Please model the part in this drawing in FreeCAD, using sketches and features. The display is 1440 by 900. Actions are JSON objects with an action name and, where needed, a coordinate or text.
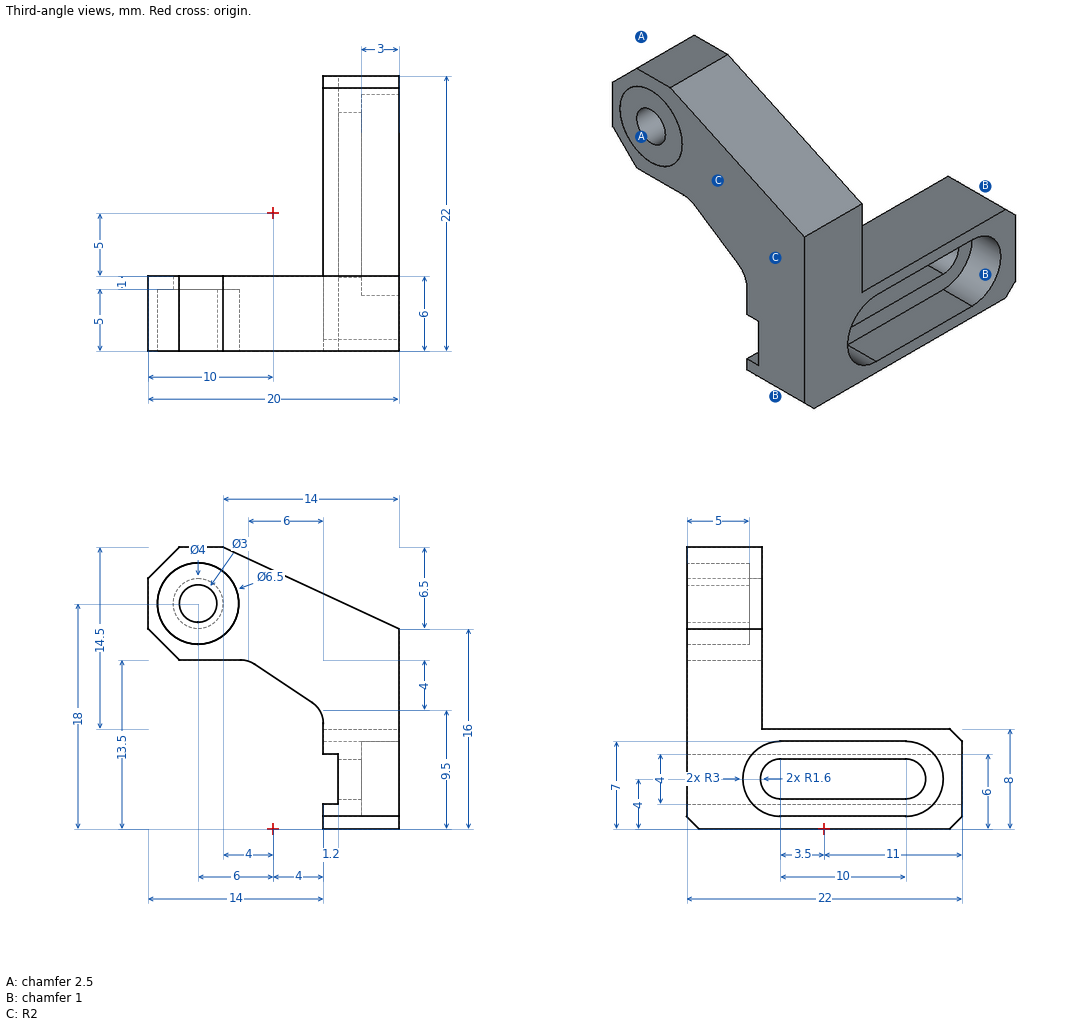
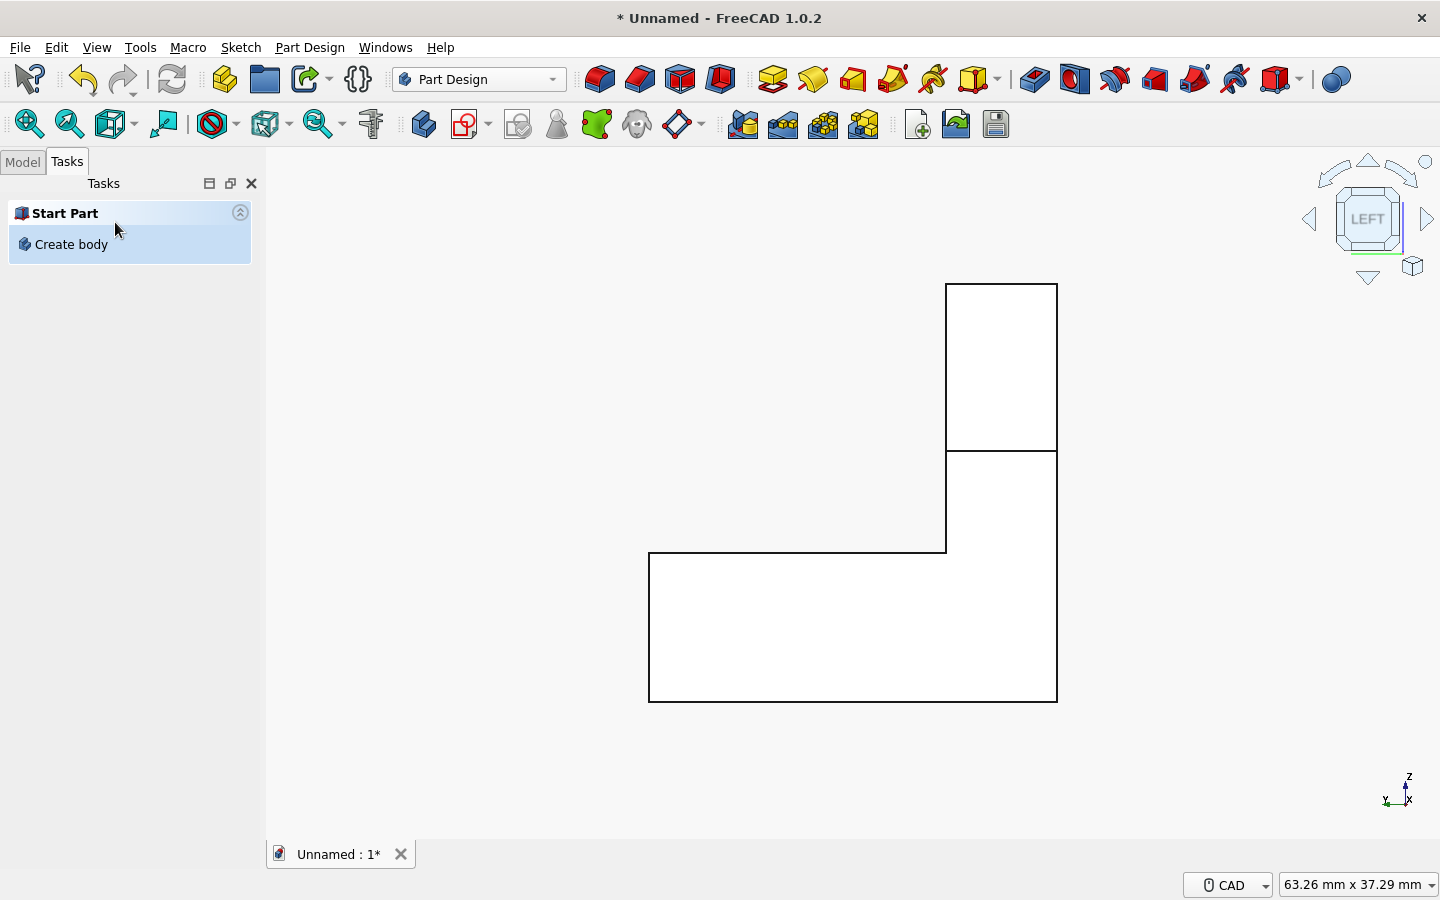
{"action": "left_click", "coordinate": [970, 611]}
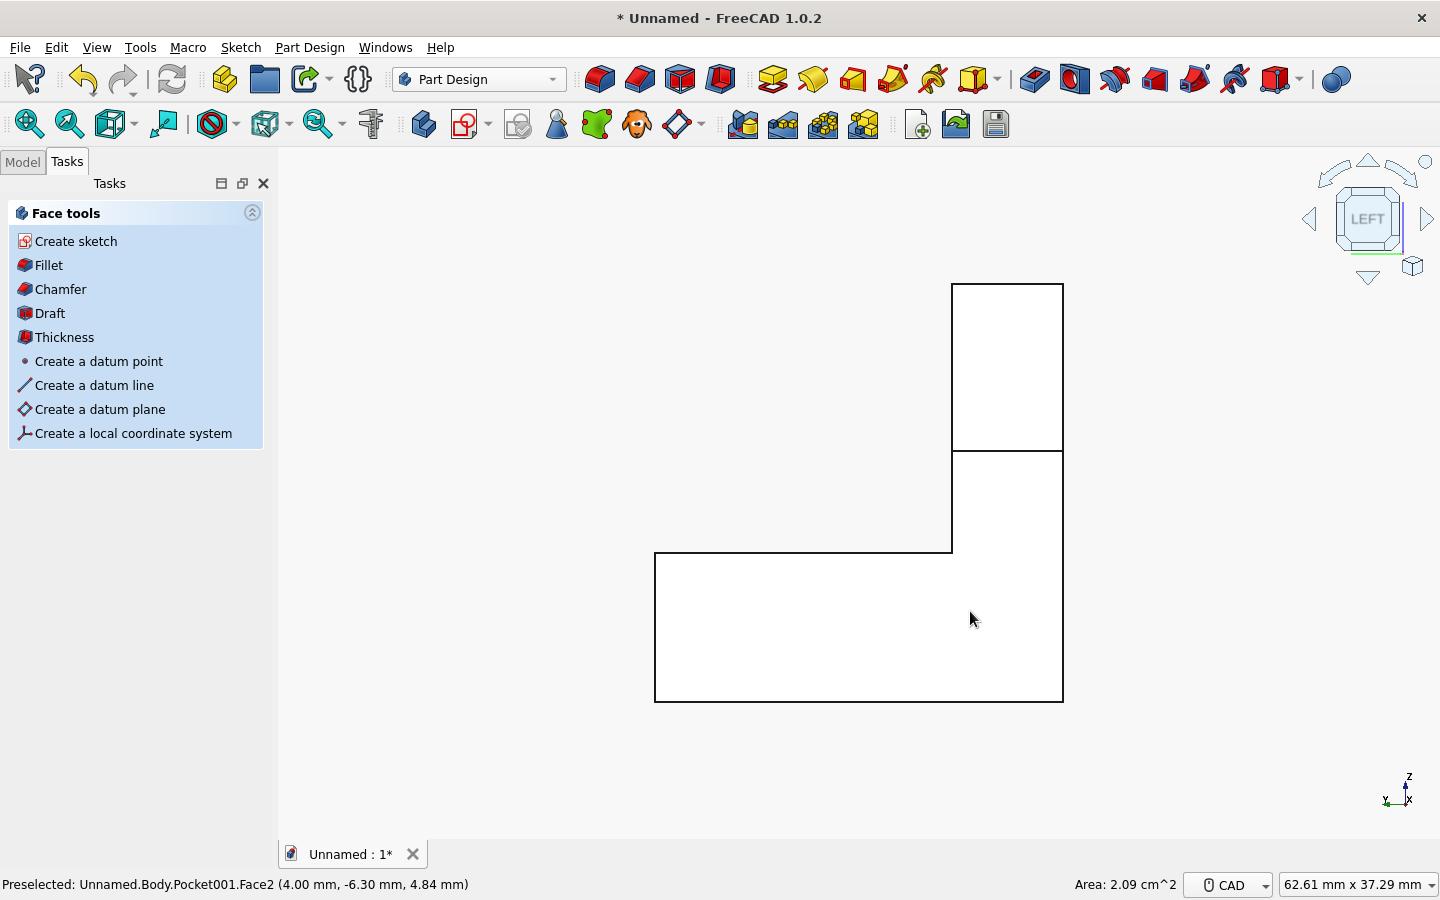
{"action": "left_click", "coordinate": [464, 124]}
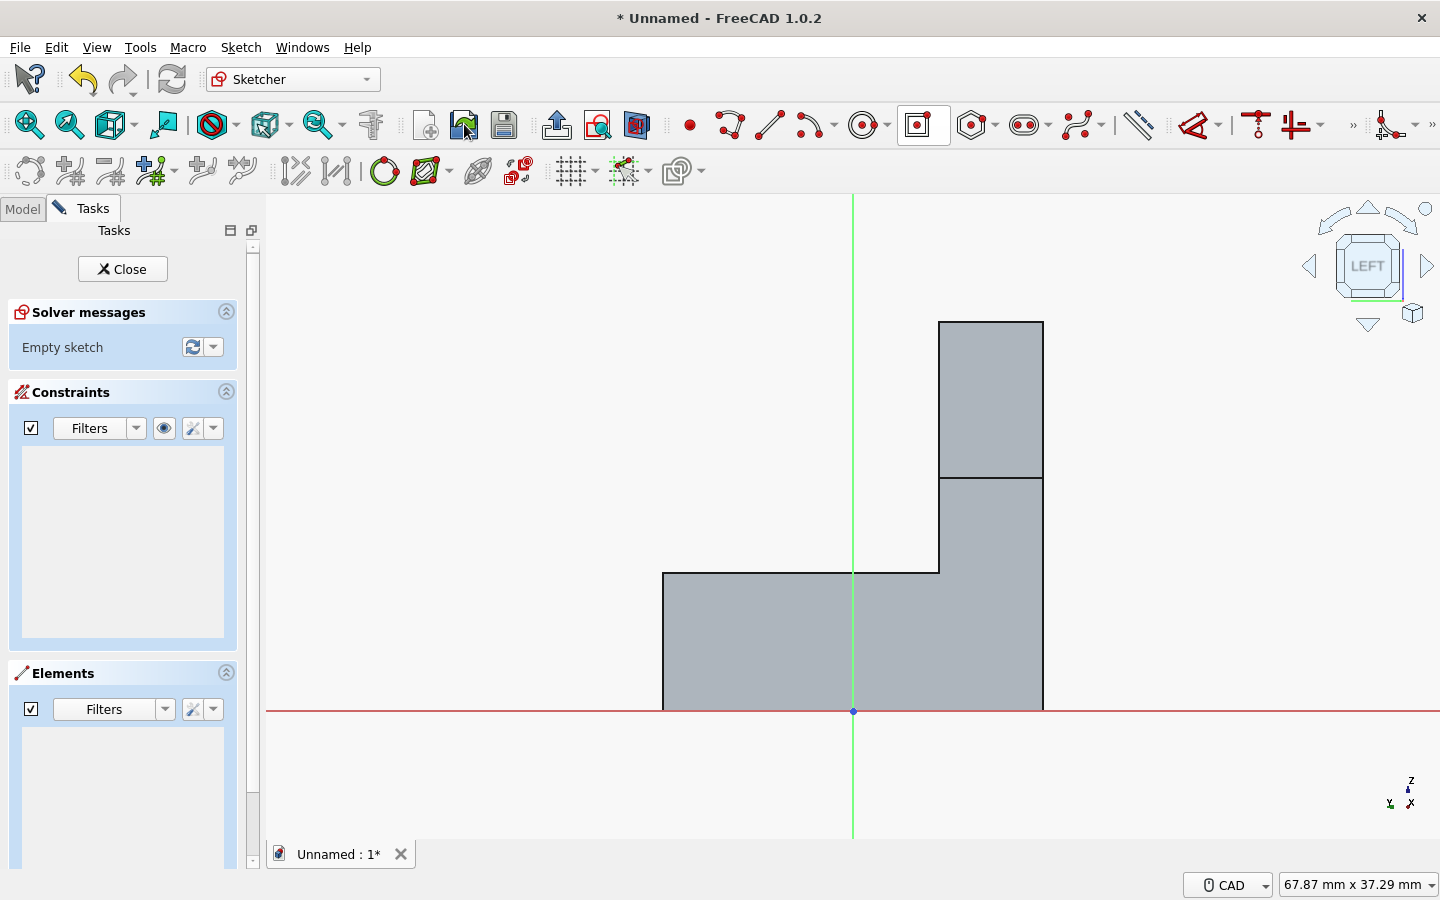
{"action": "left_click", "coordinate": [638, 126]}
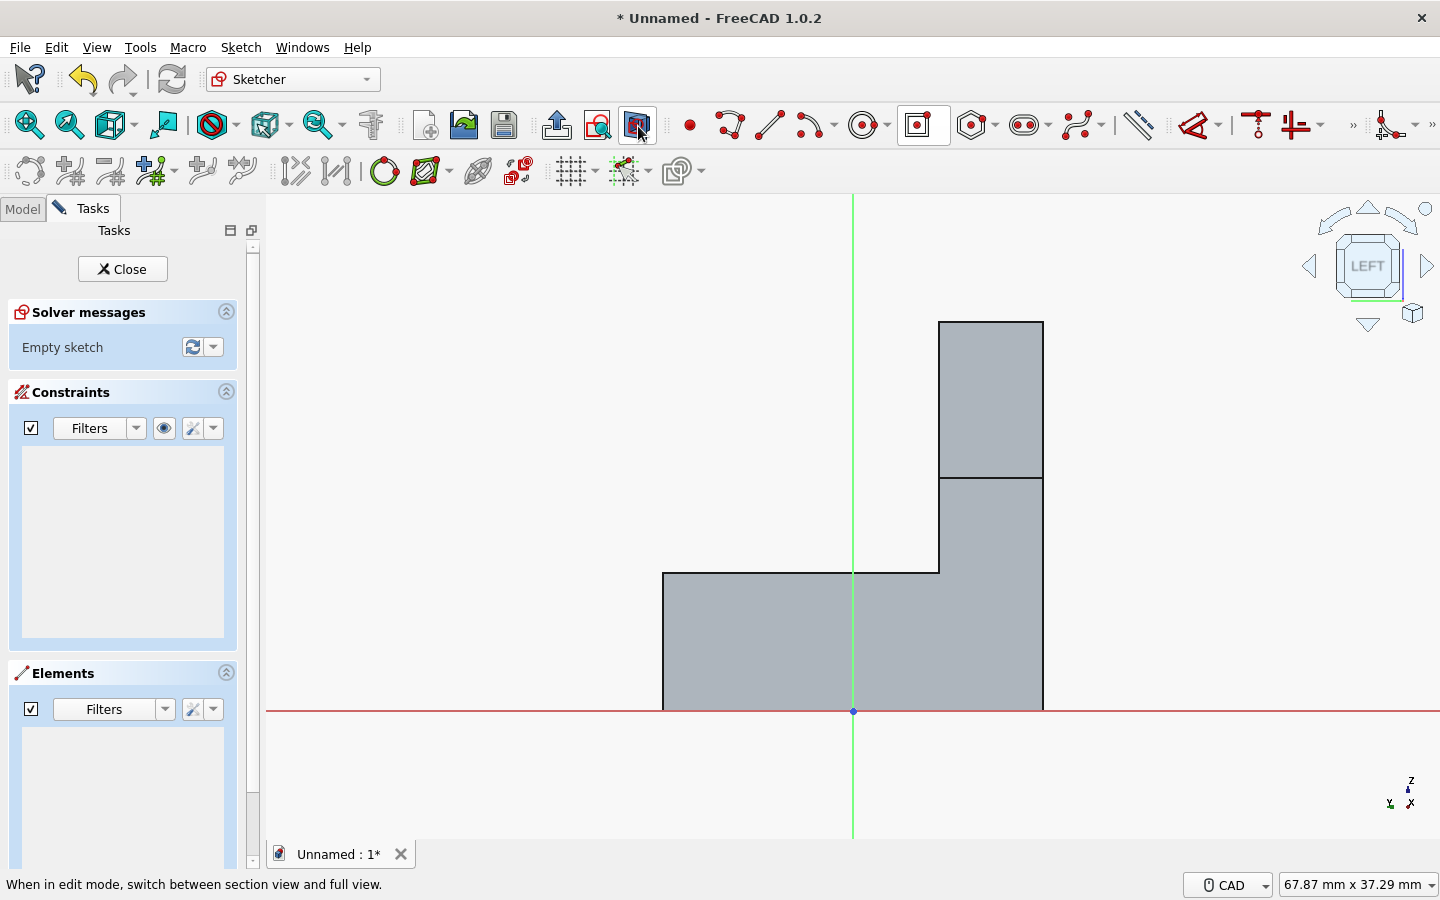
{"action": "scroll", "coordinate": [936, 811], "scroll_direction": "up", "scroll_amount": 3}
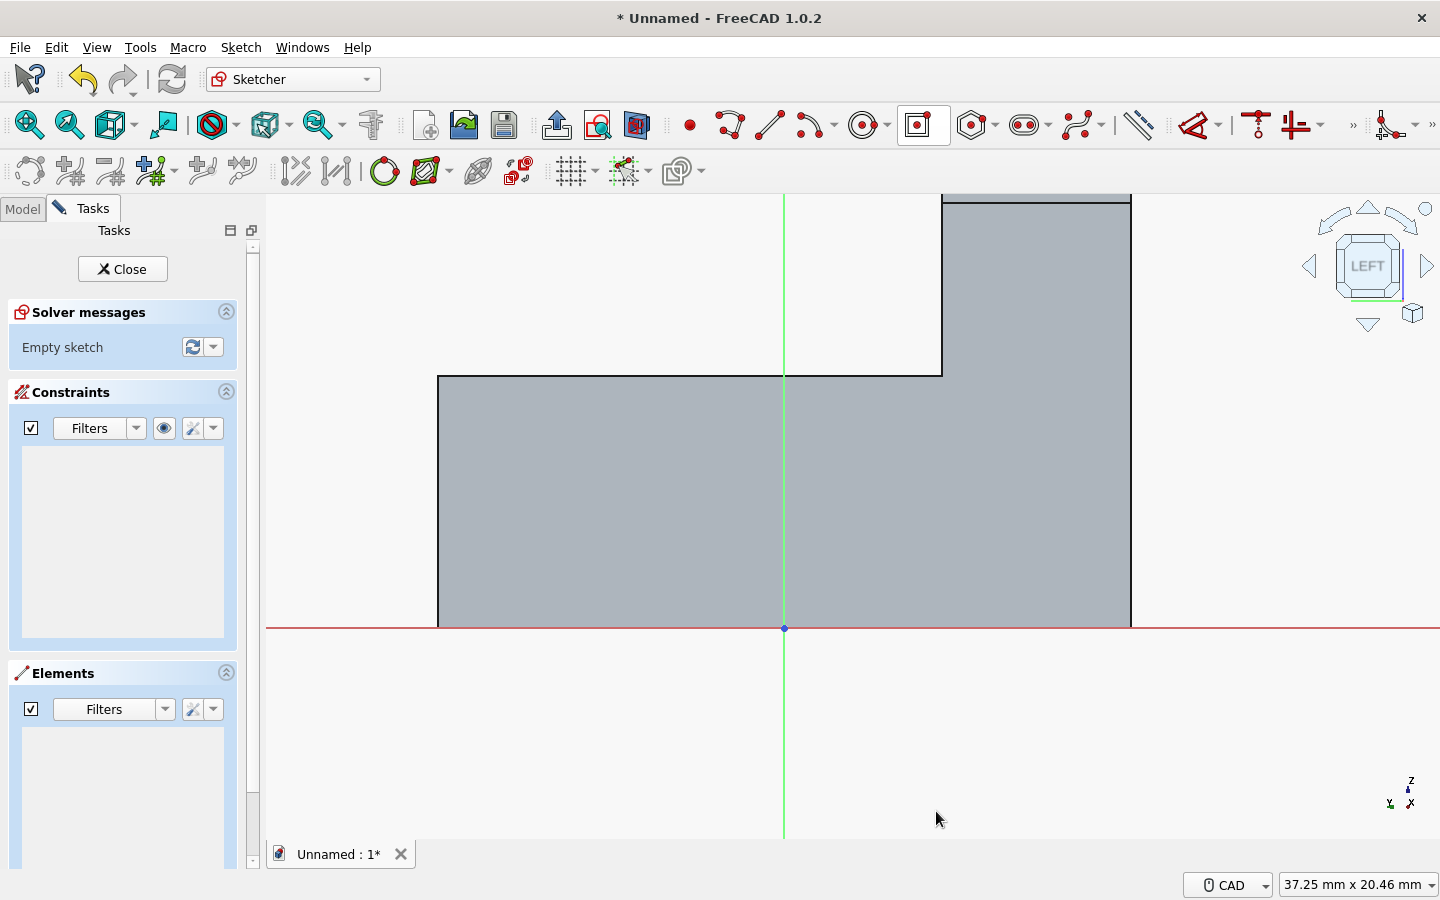
{"action": "key", "text": "g r"}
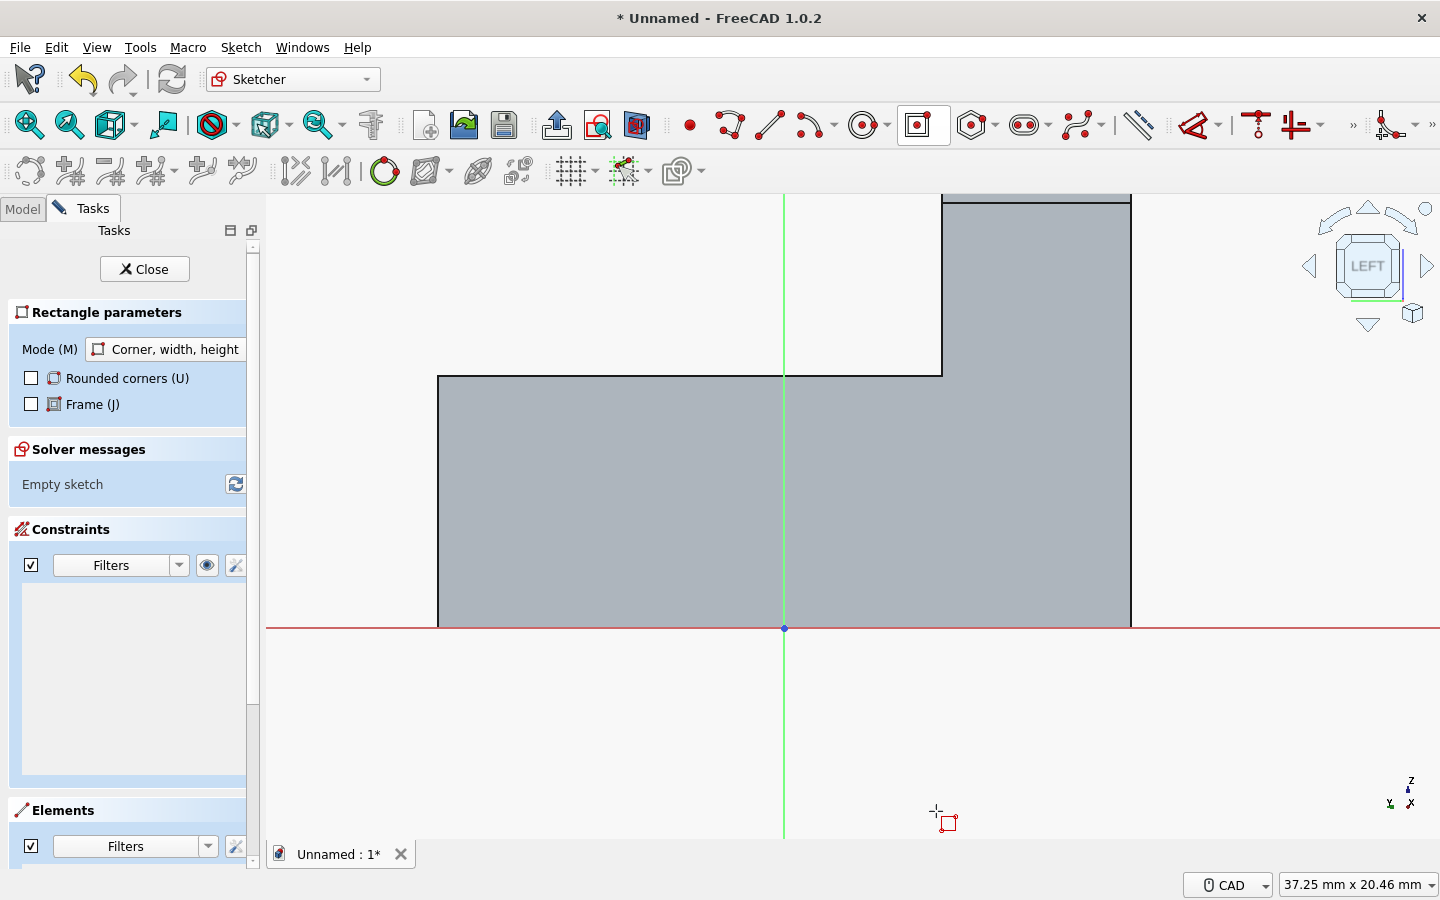
{"action": "left_click", "coordinate": [438, 439]}
{"action": "mouse_move", "coordinate": [1131, 565]}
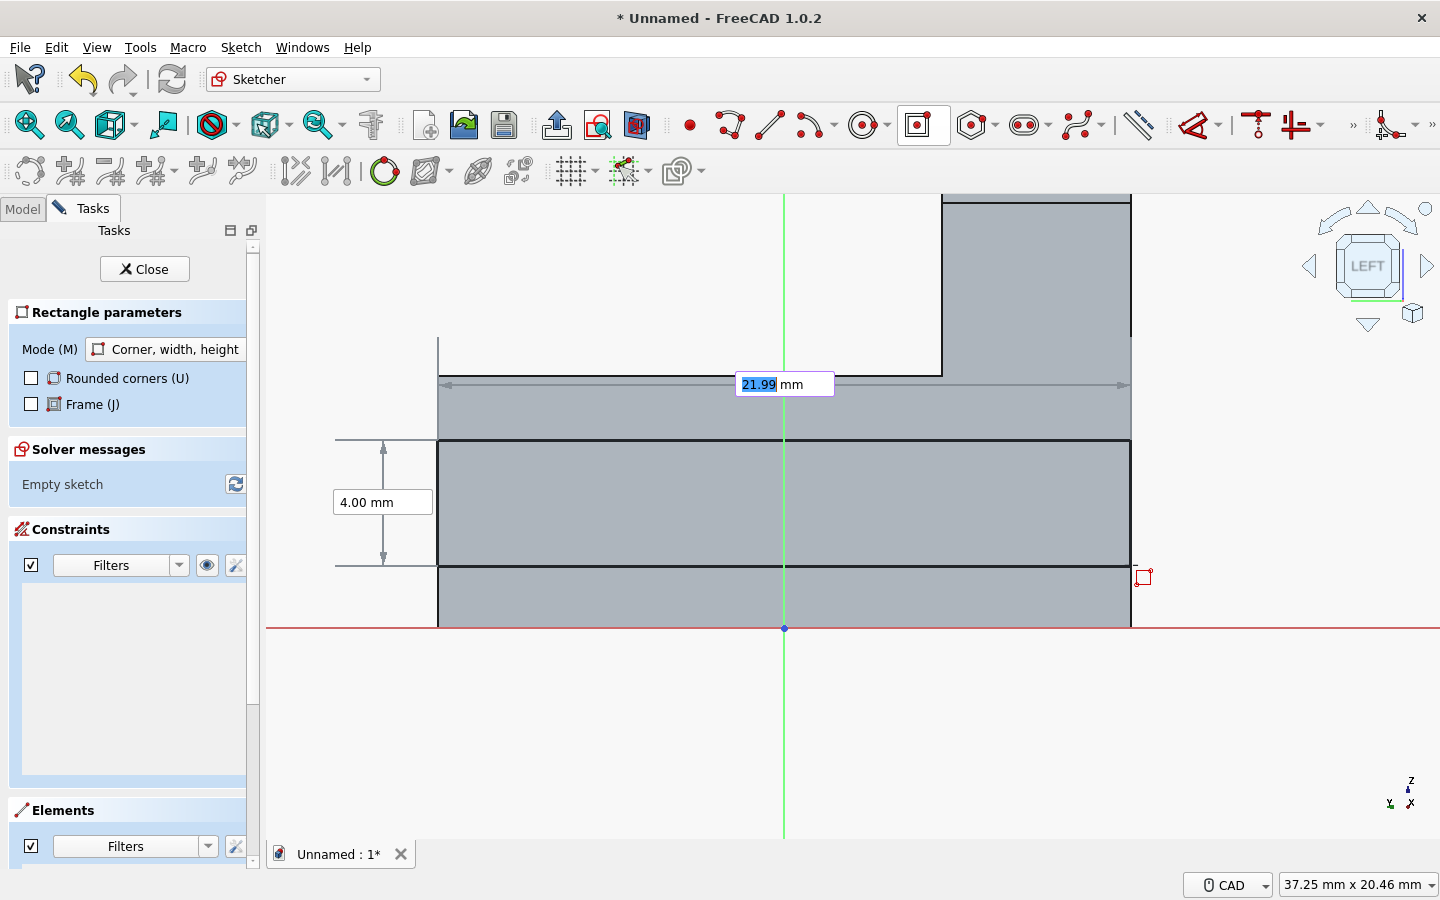
{"action": "type", "text": "22"}
{"action": "key", "text": "Tab"}
{"action": "type", "text": "4"}
{"action": "key", "text": "Return"}
{"action": "key", "text": "Escape"}